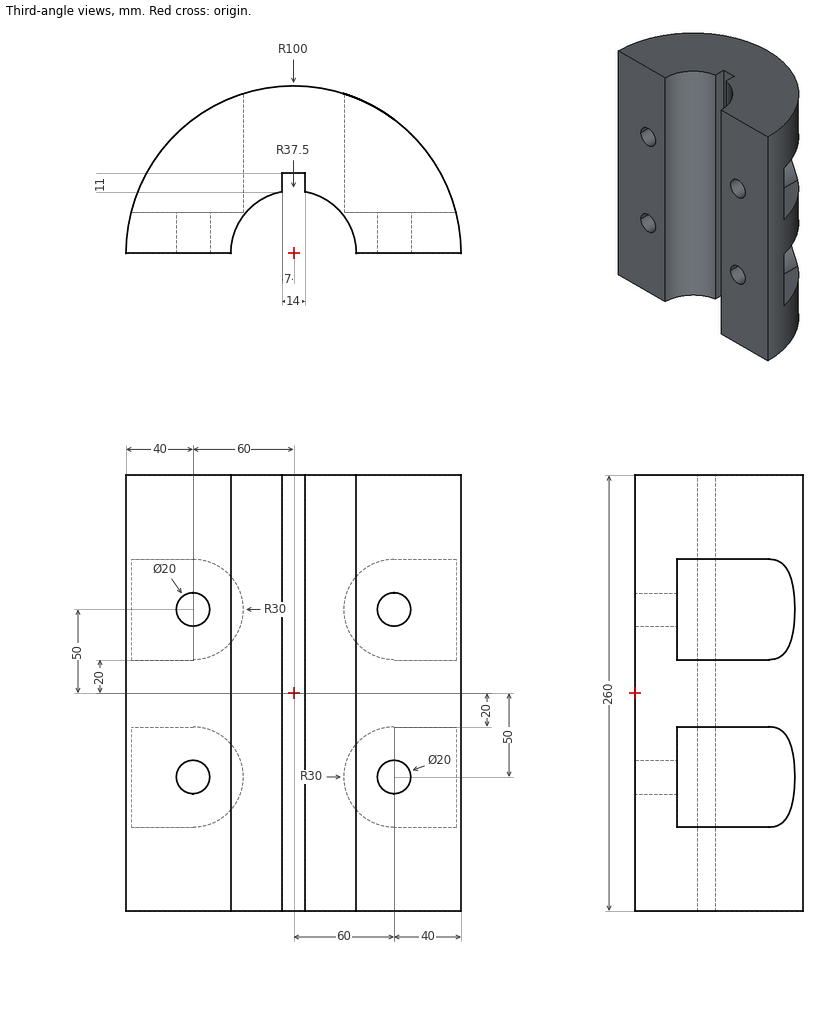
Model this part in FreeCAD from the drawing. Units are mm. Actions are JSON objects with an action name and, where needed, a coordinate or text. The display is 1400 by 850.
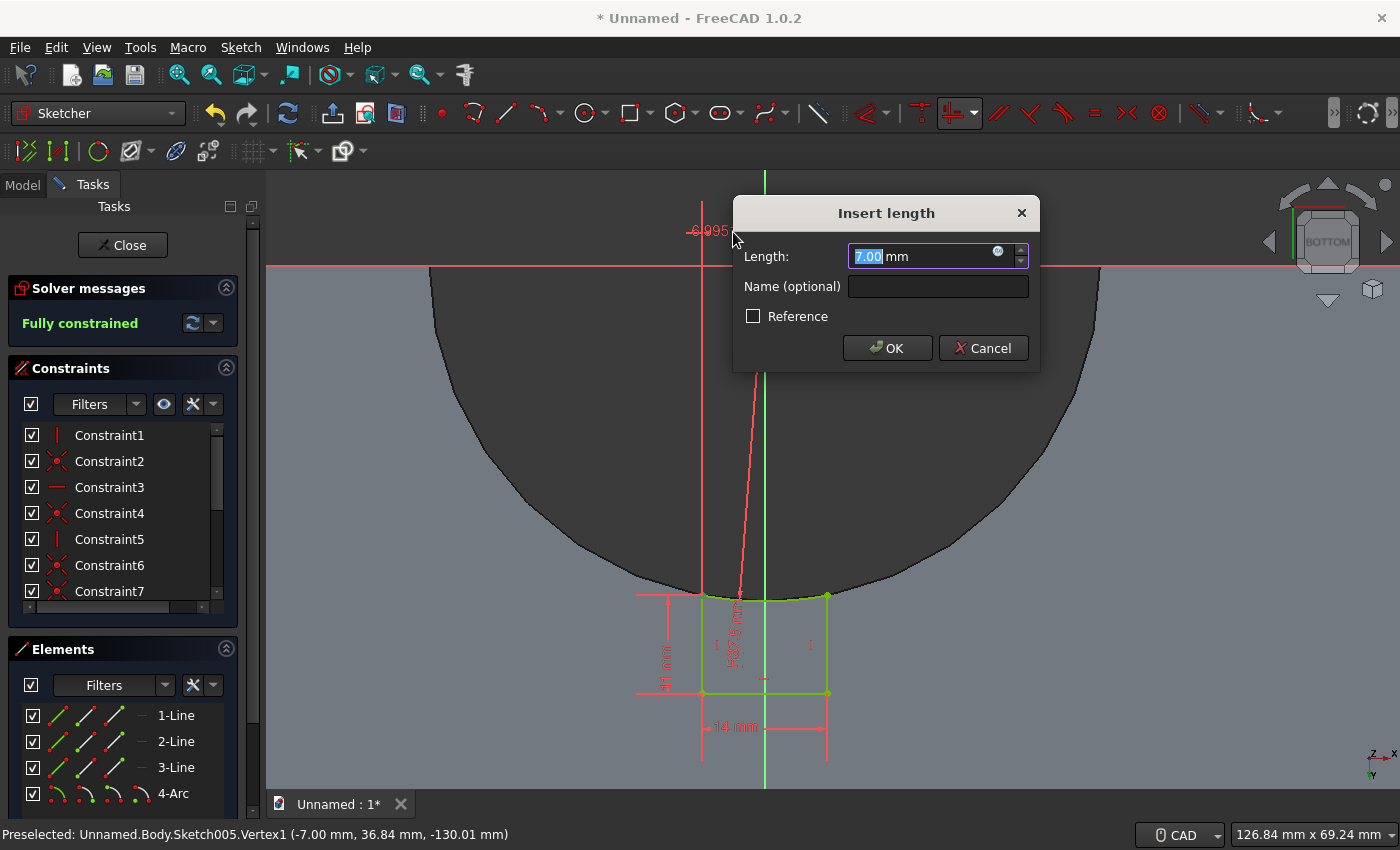
{"action": "type", "text": "7"}
{"action": "key", "text": "Return"}
{"action": "key", "text": "Escape"}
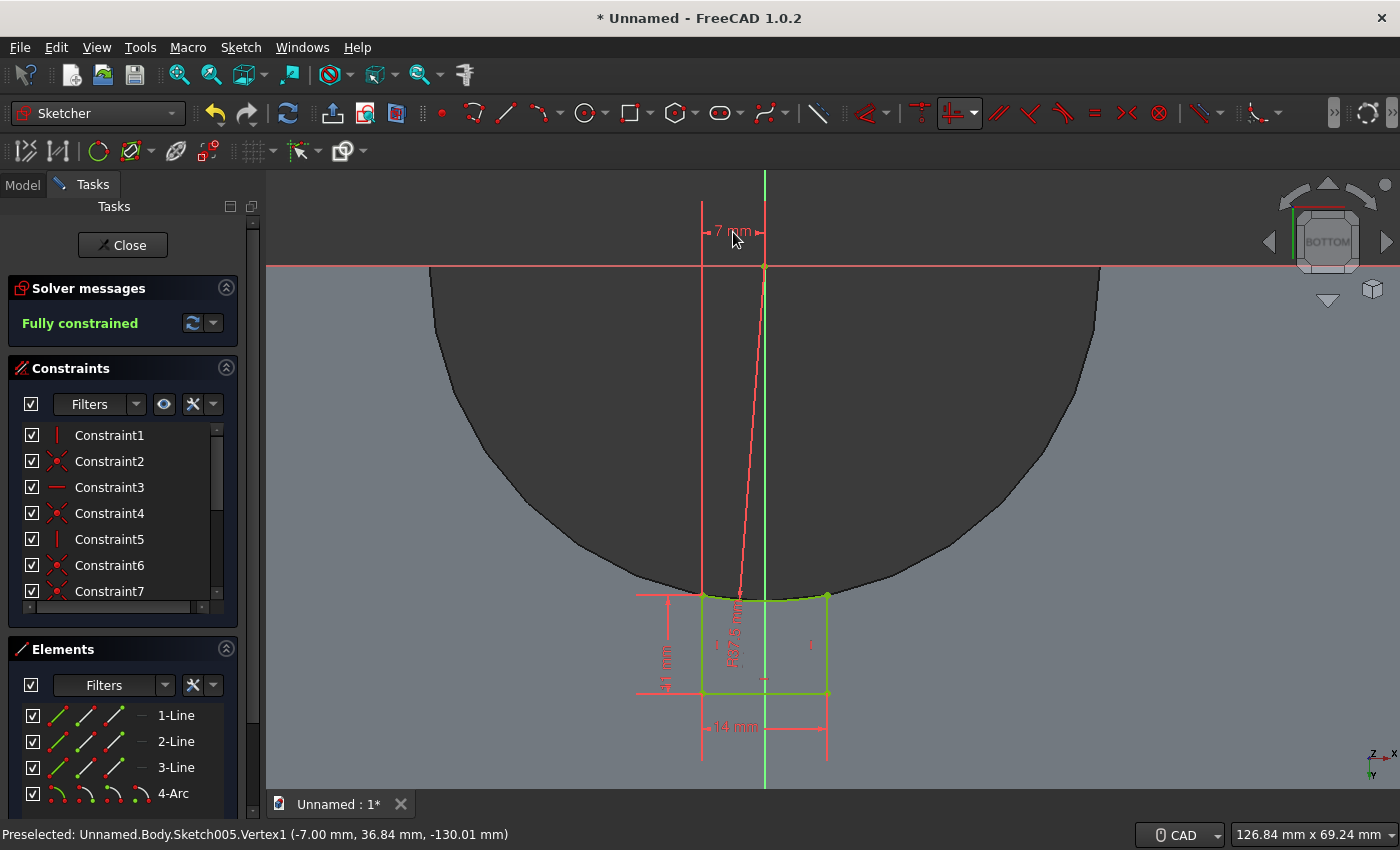
{"action": "left_click", "coordinate": [123, 245]}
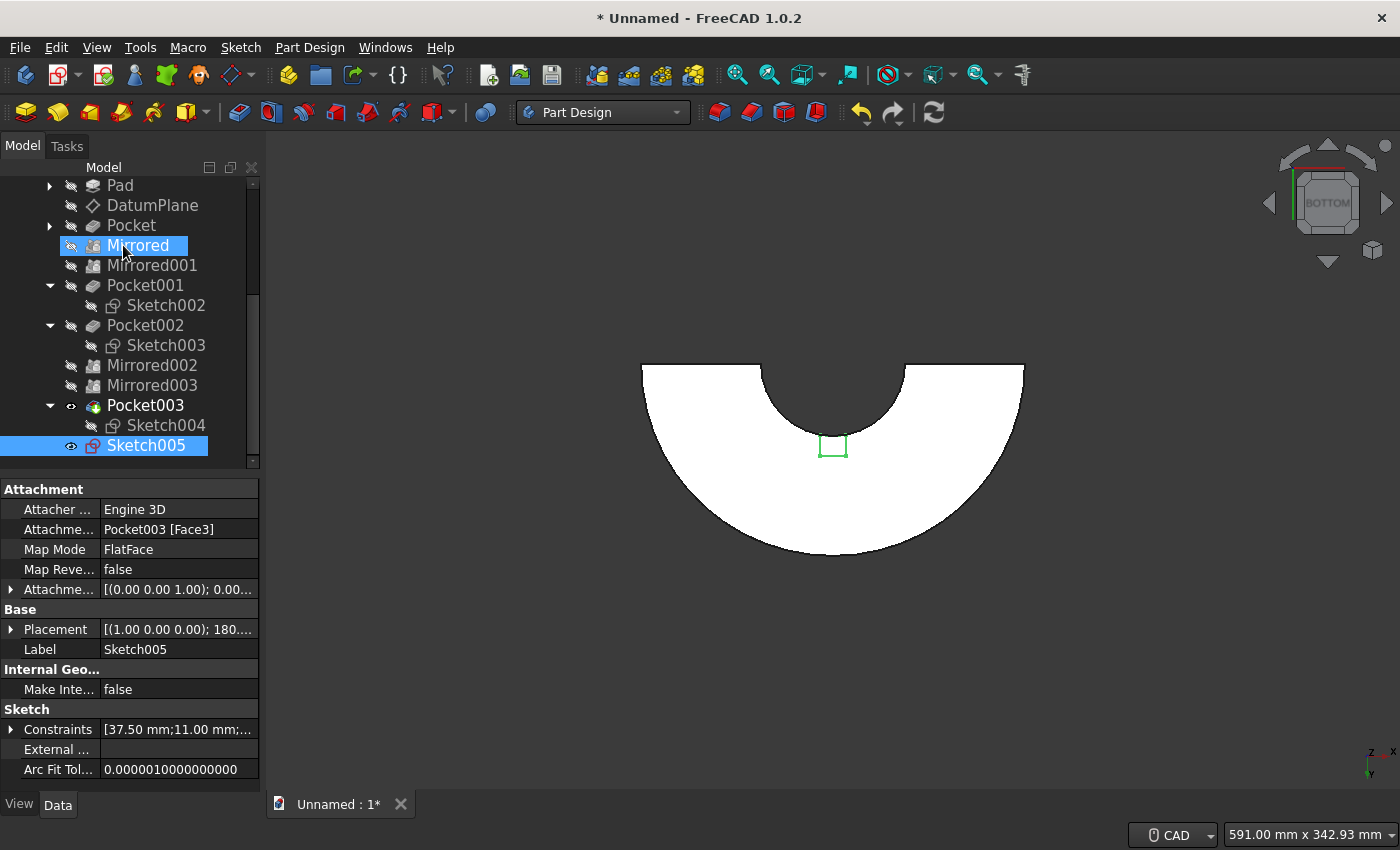
{"action": "left_click", "coordinate": [240, 112]}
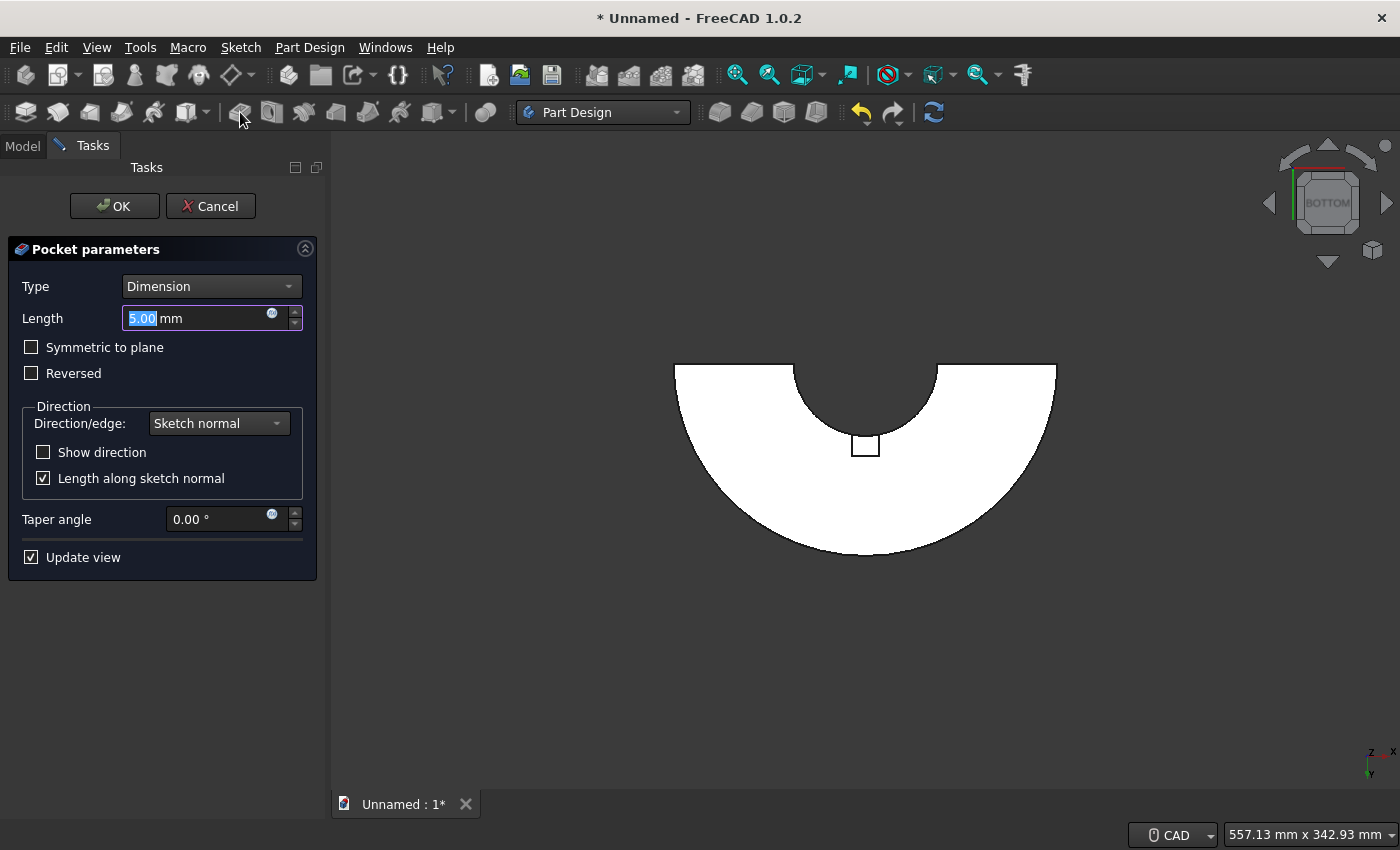
{"action": "left_click", "coordinate": [212, 286]}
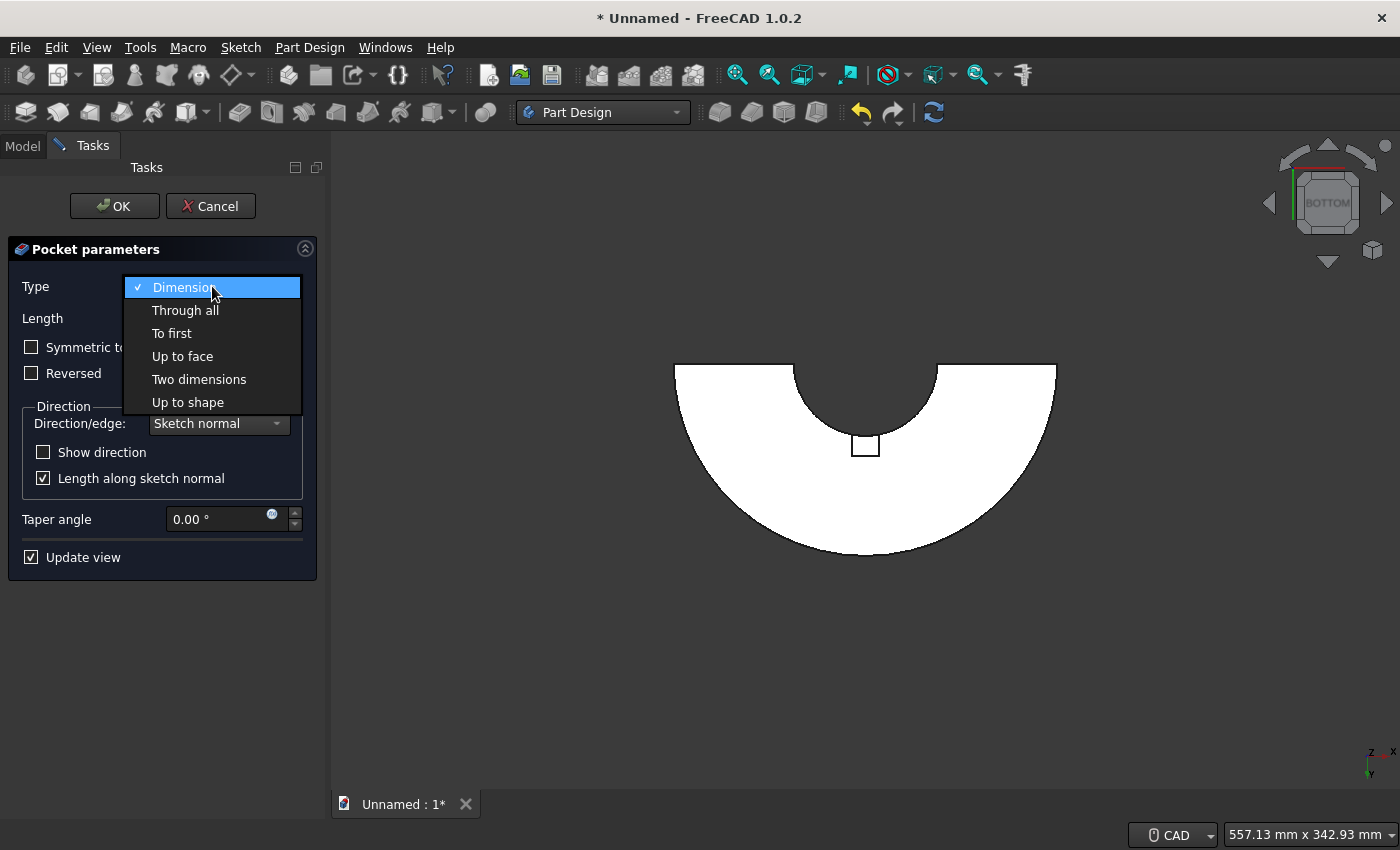
{"action": "left_click", "coordinate": [212, 310]}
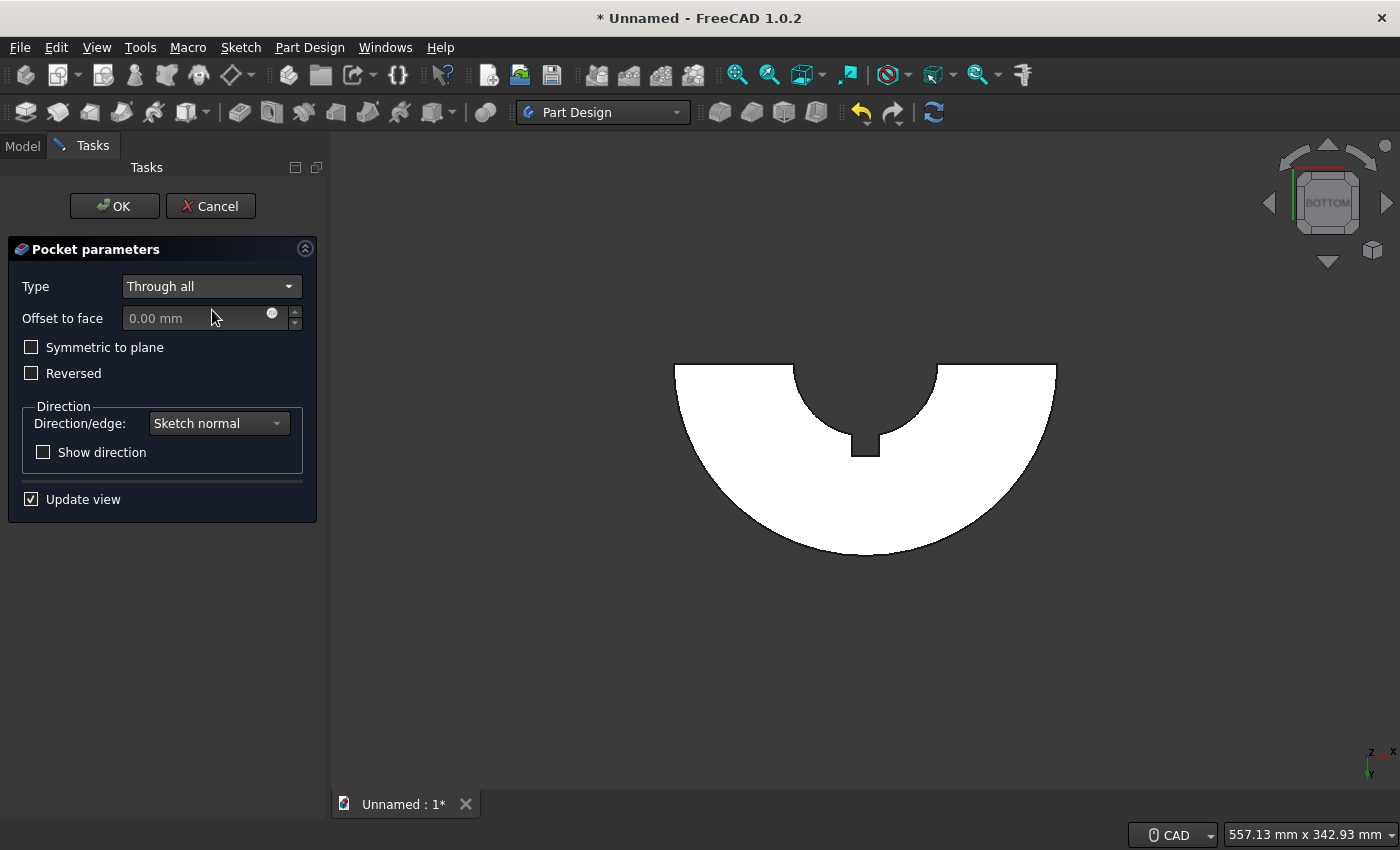
{"action": "left_click", "coordinate": [115, 206]}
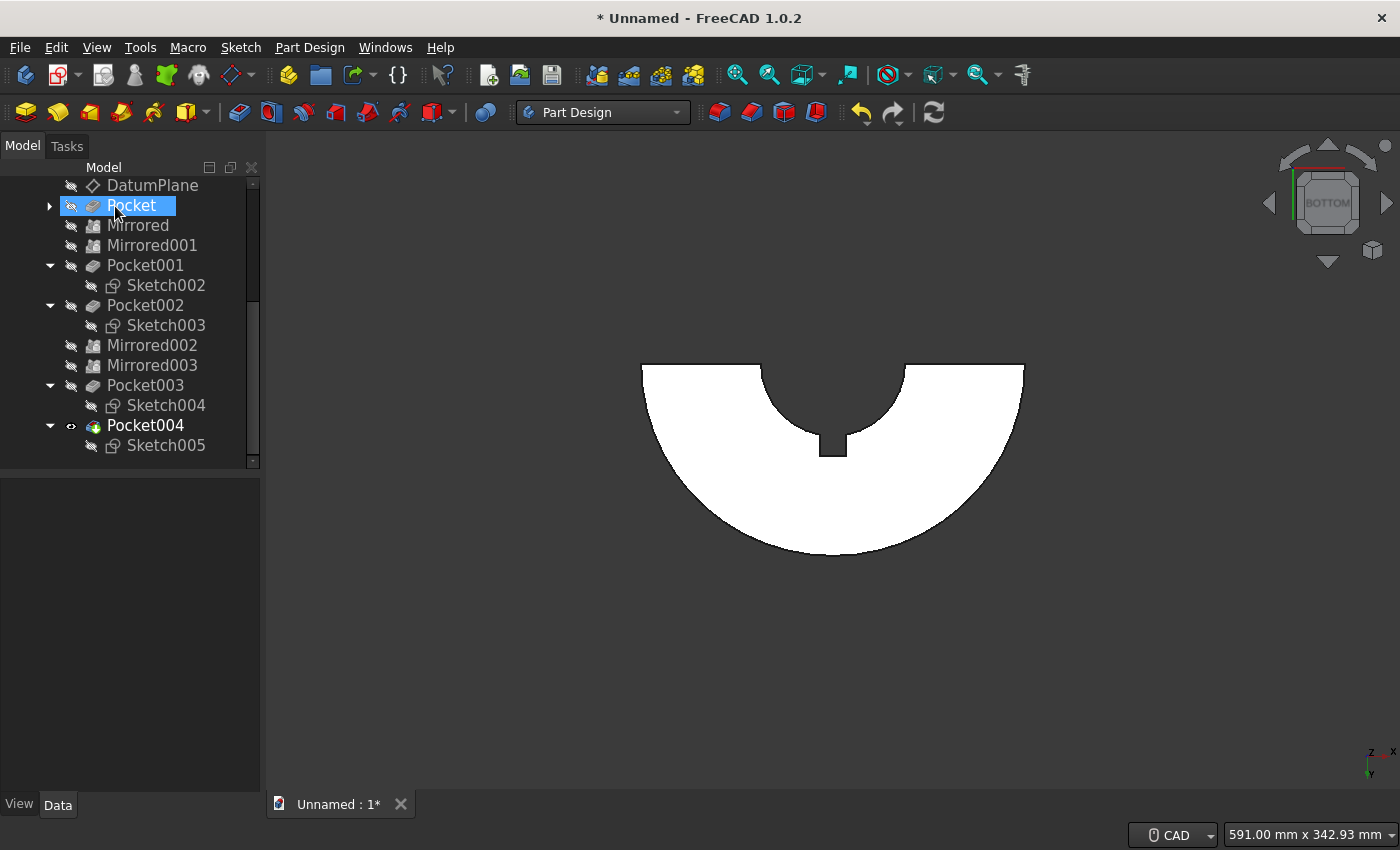
{"action": "key", "text": "0"}